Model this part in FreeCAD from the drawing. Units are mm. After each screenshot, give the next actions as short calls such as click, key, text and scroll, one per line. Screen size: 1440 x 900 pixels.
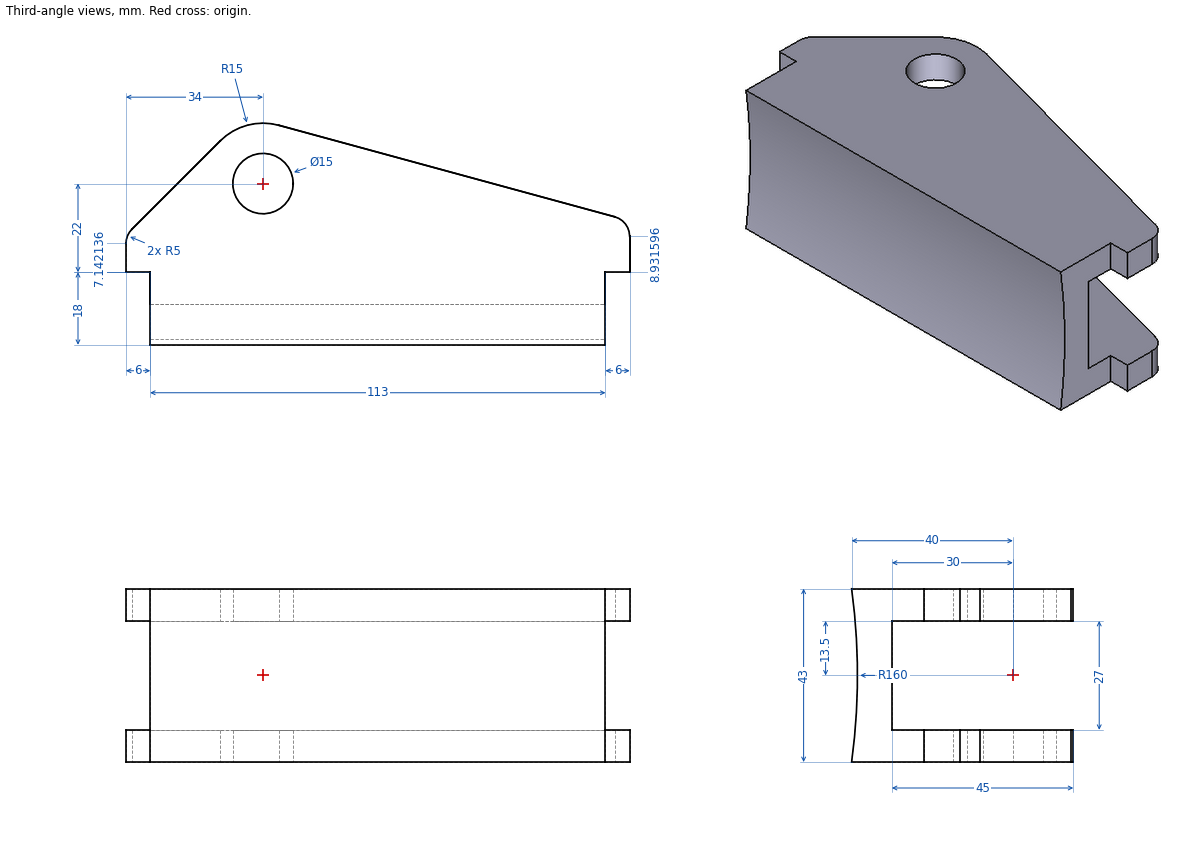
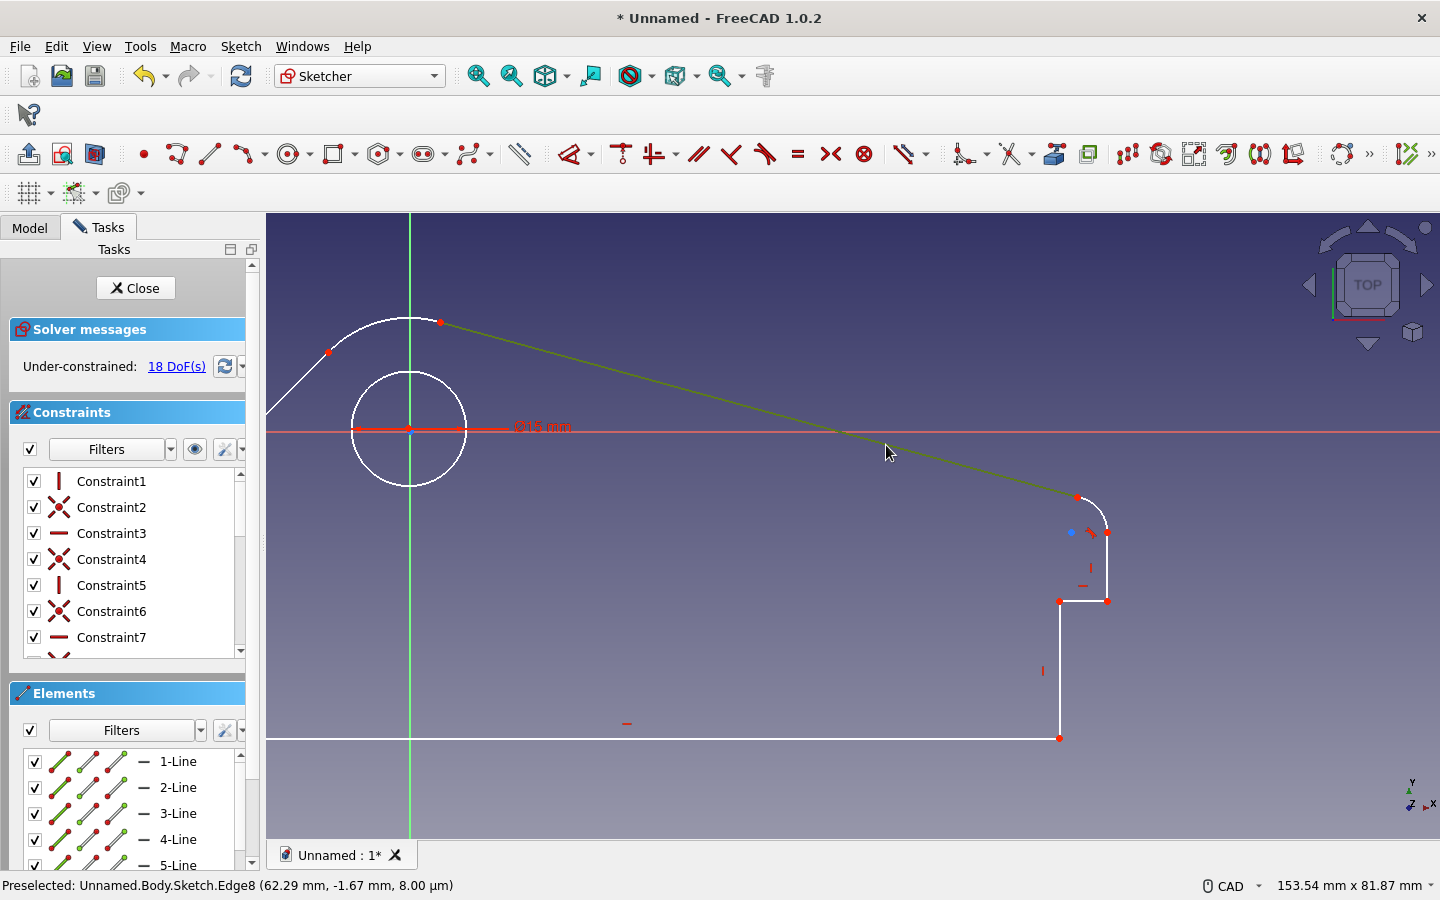
click(1104, 518)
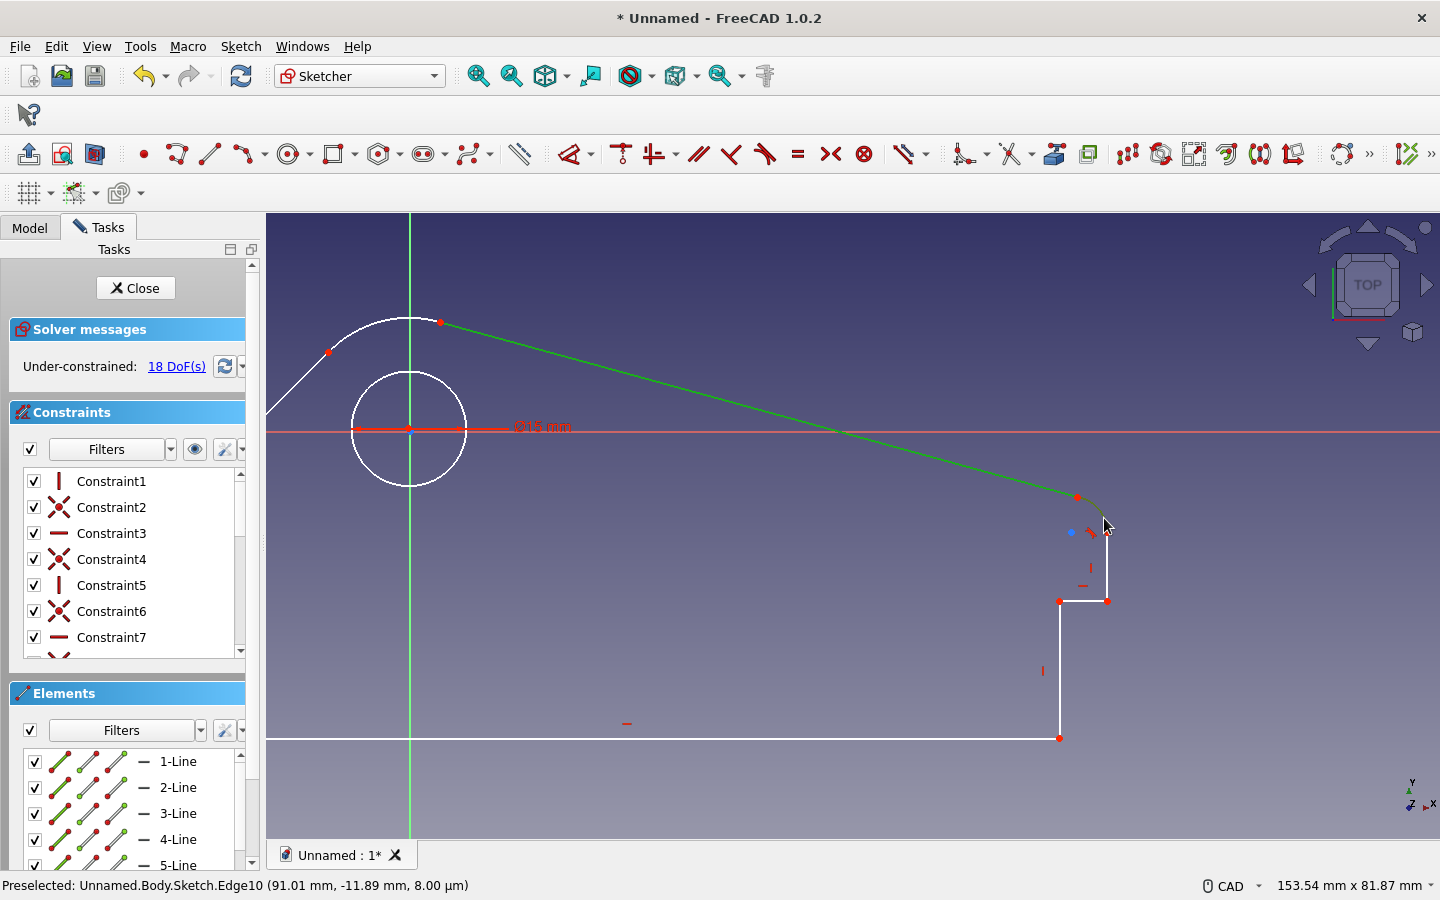
click(765, 154)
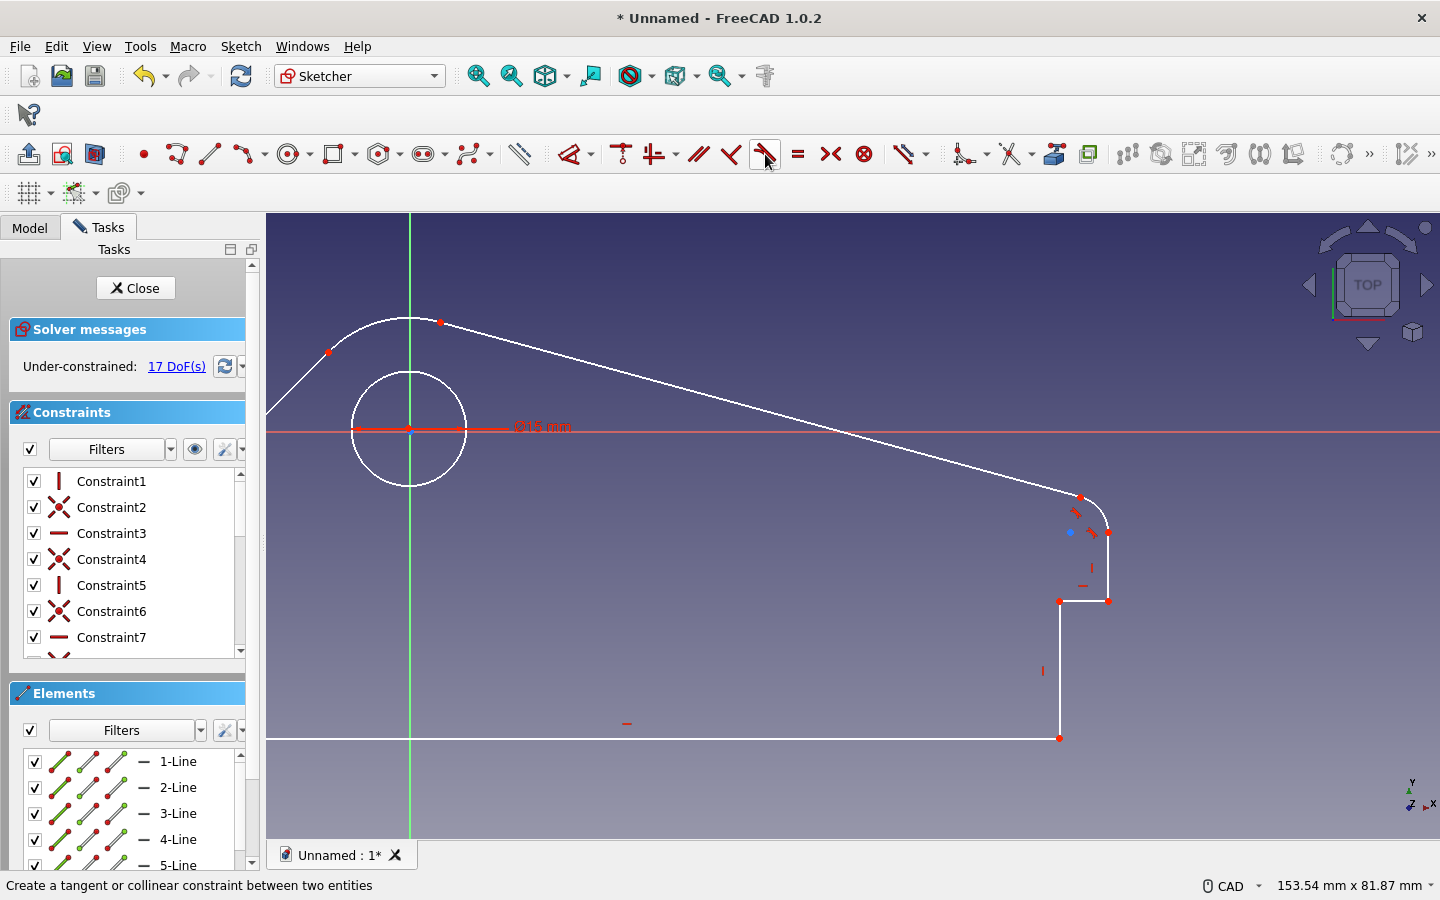
click(889, 445)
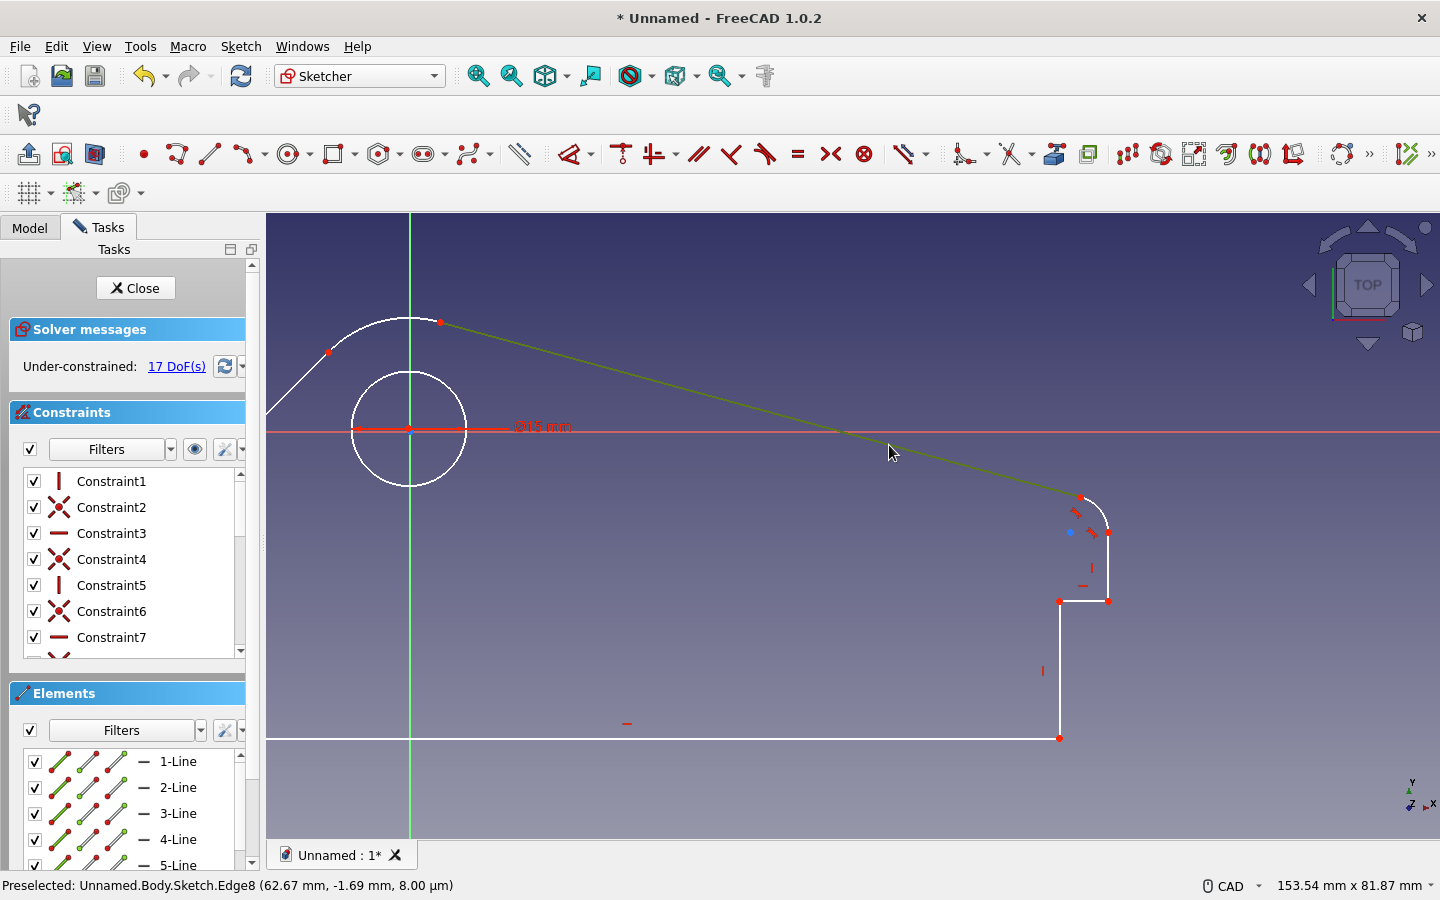
click(358, 330)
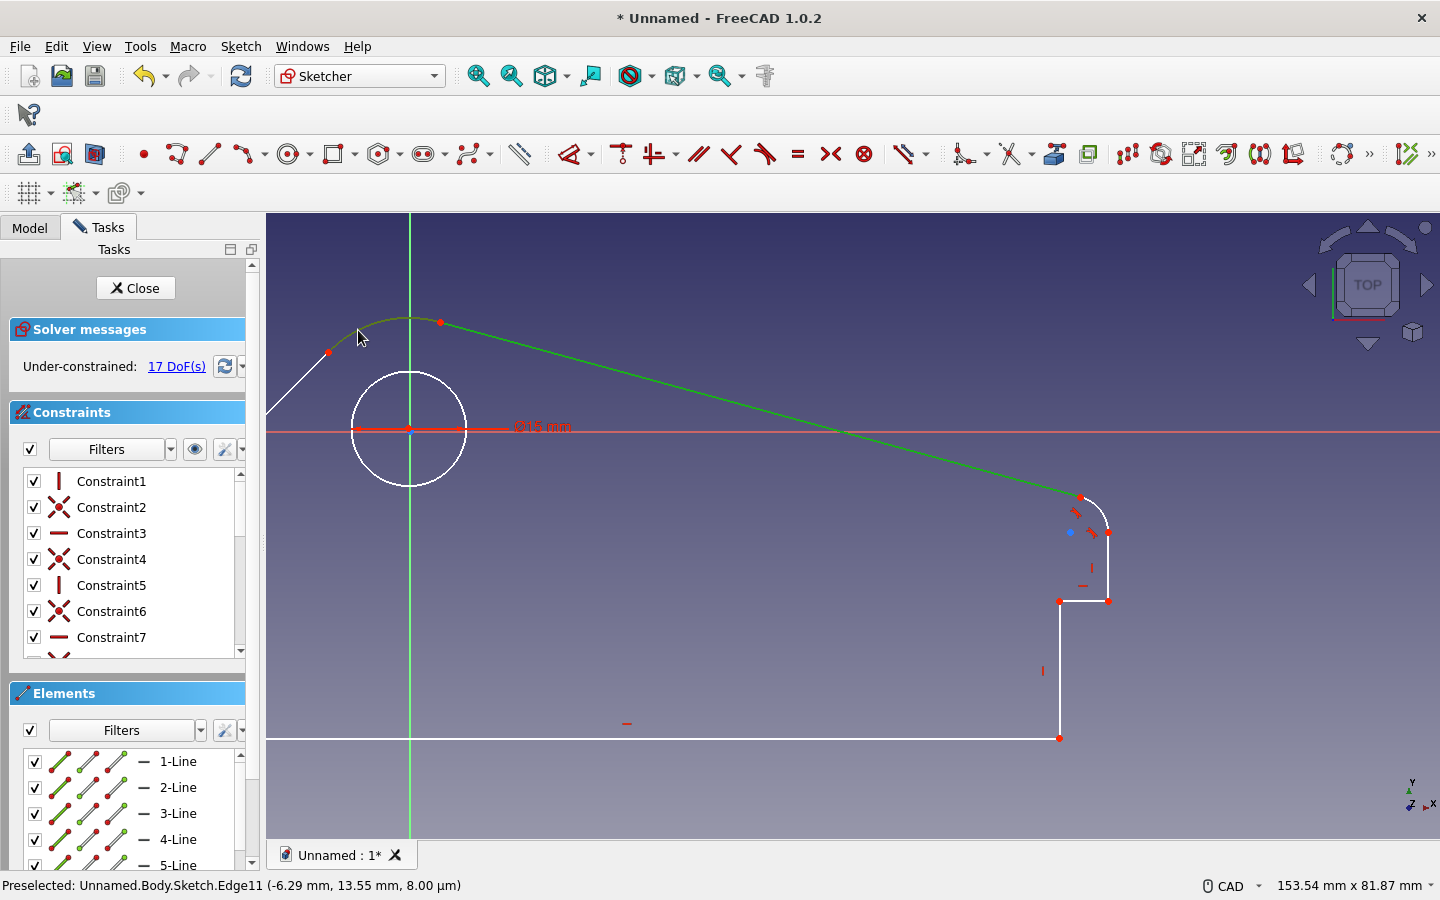
click(765, 154)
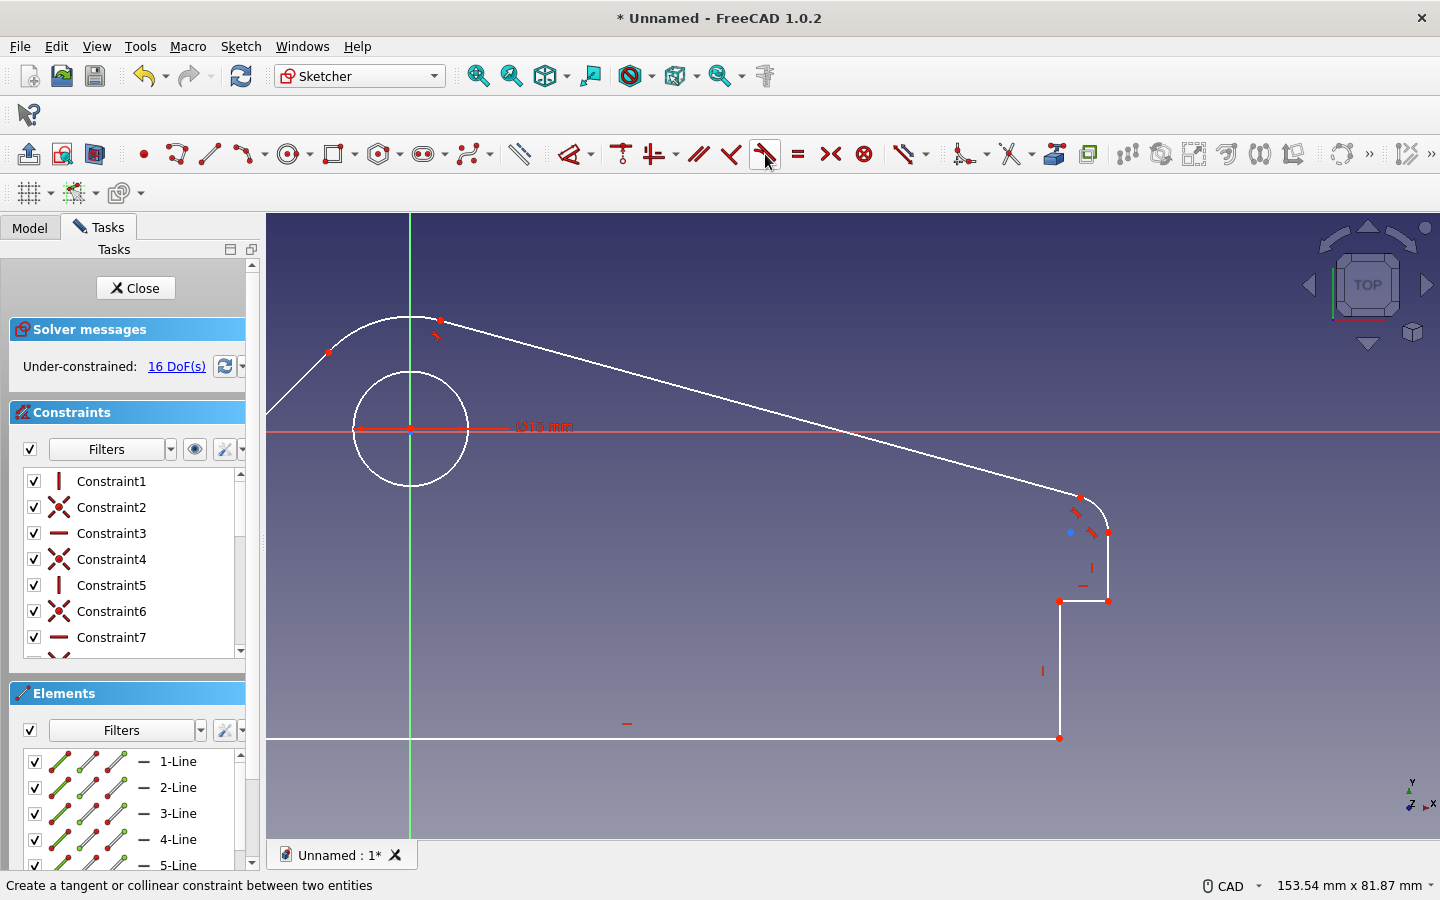
click(295, 386)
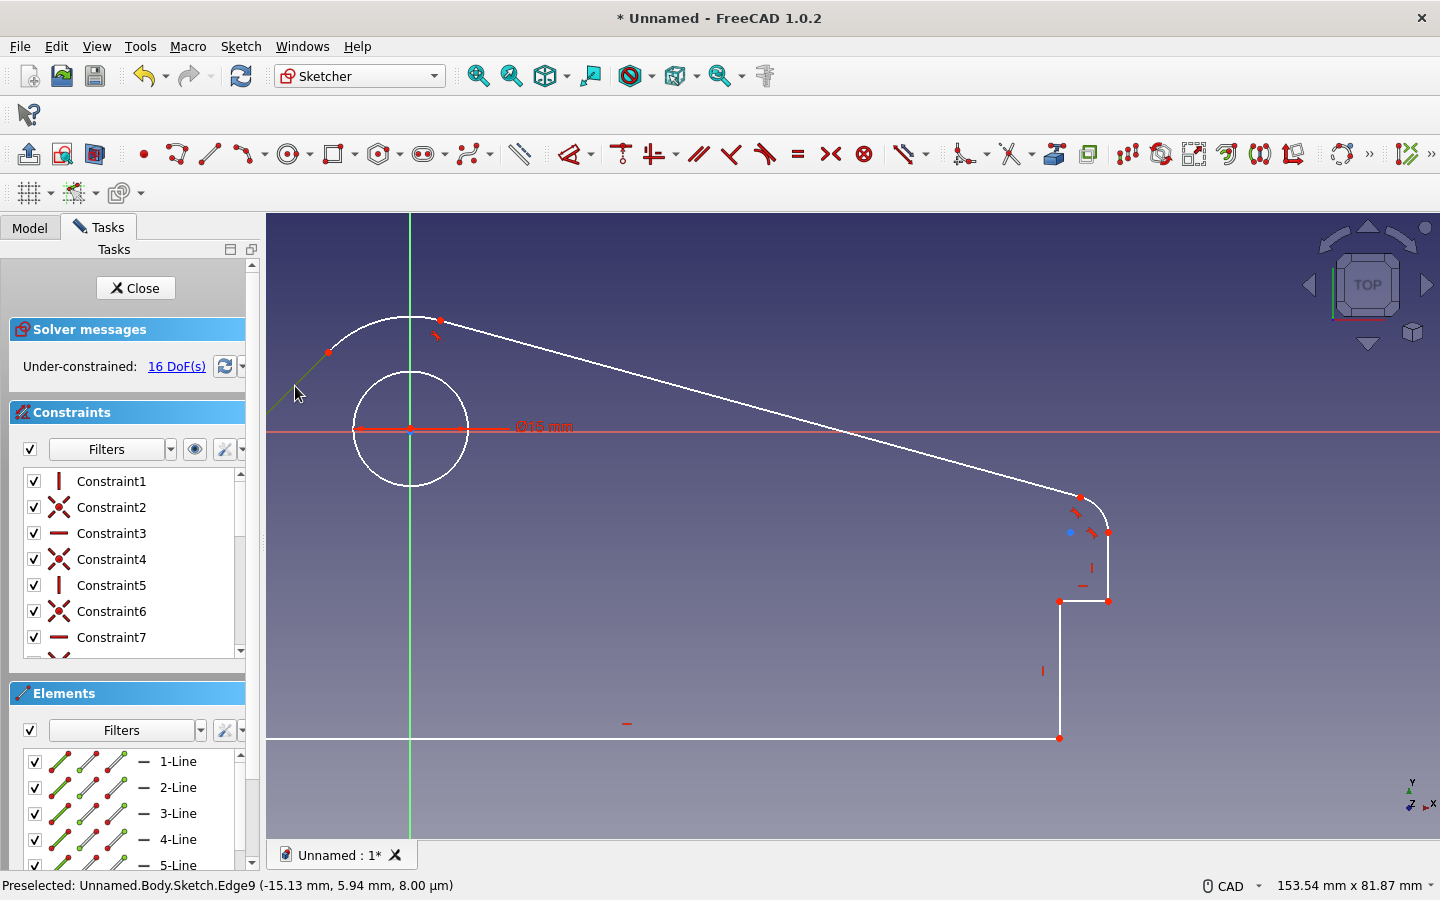
click(357, 330)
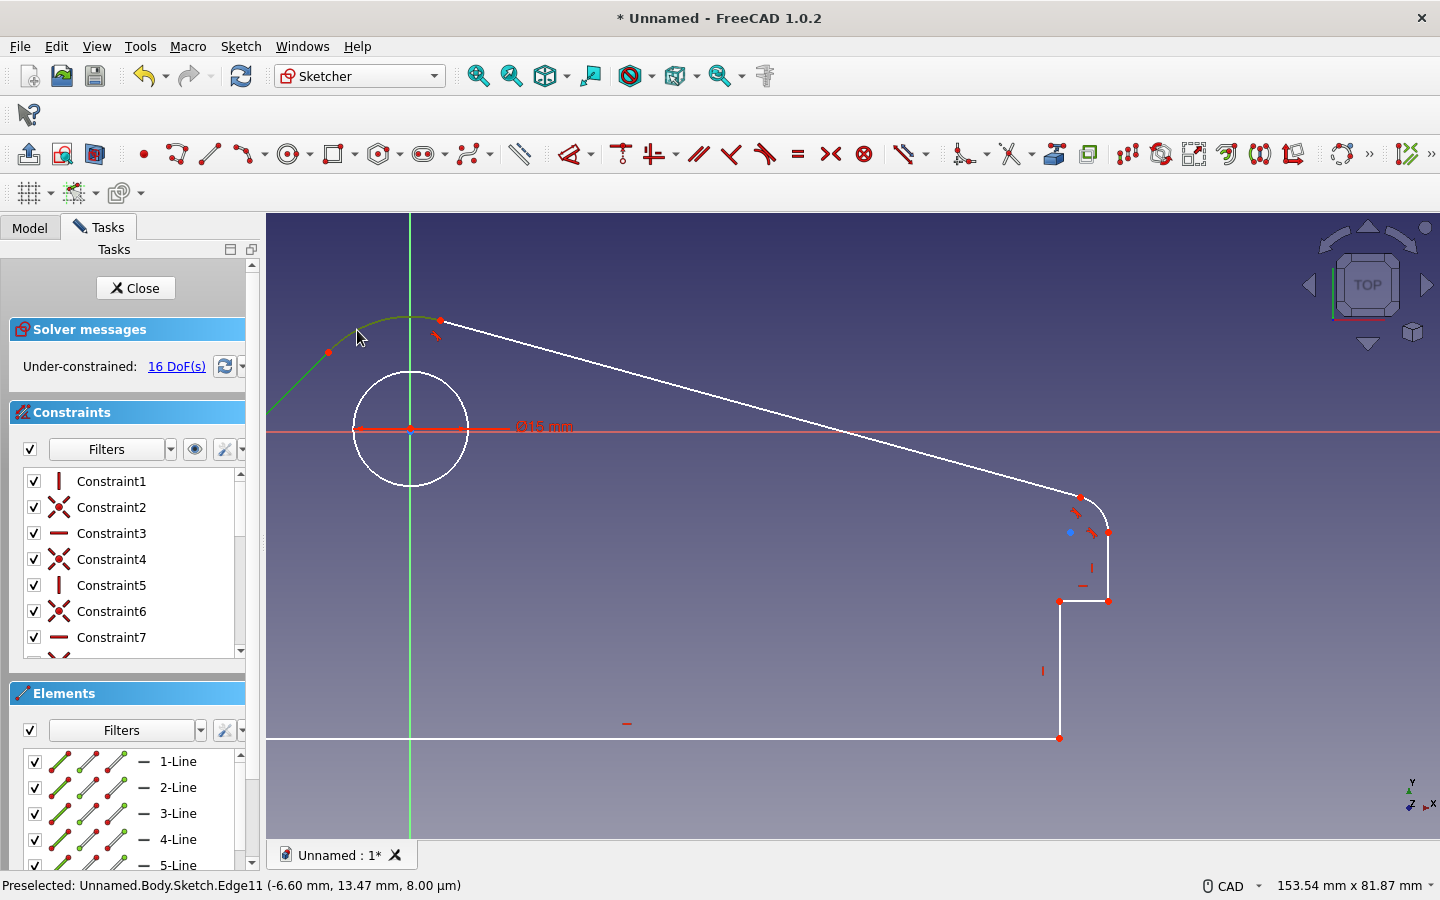
click(765, 154)